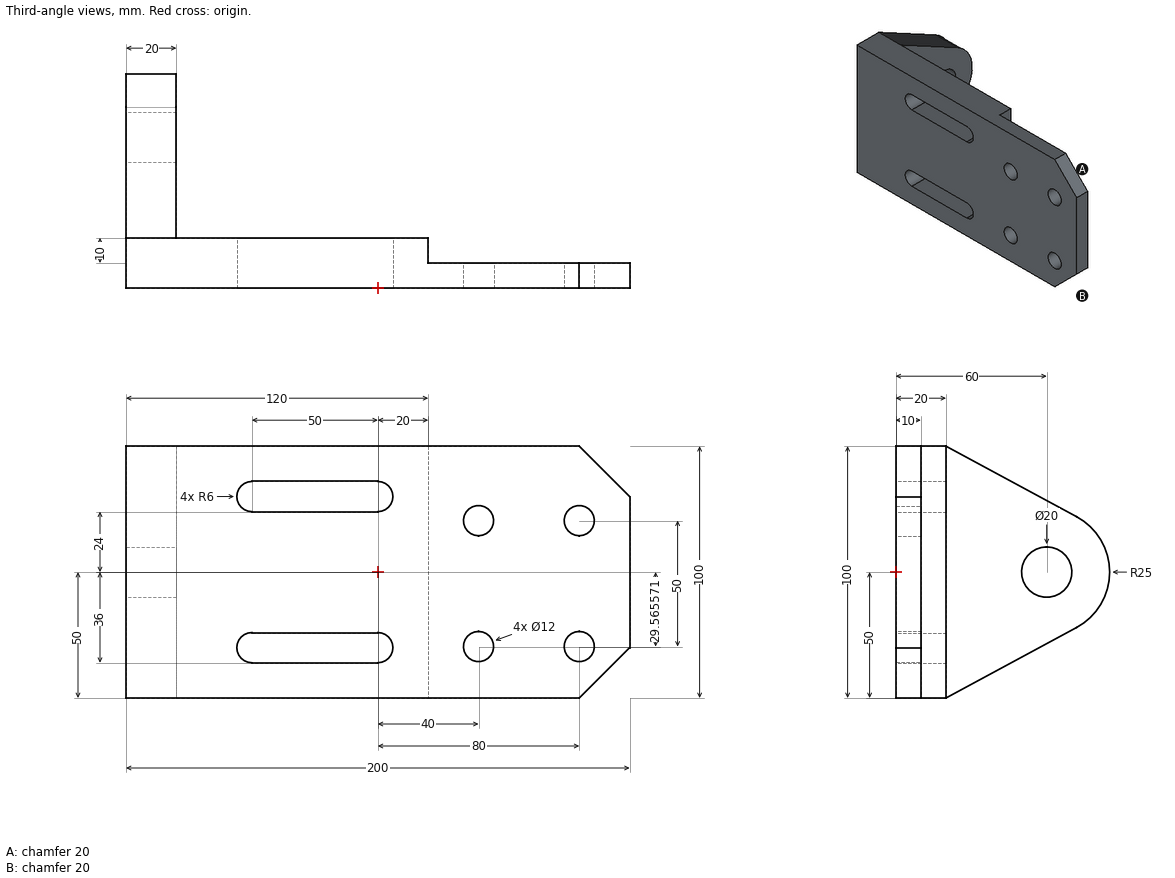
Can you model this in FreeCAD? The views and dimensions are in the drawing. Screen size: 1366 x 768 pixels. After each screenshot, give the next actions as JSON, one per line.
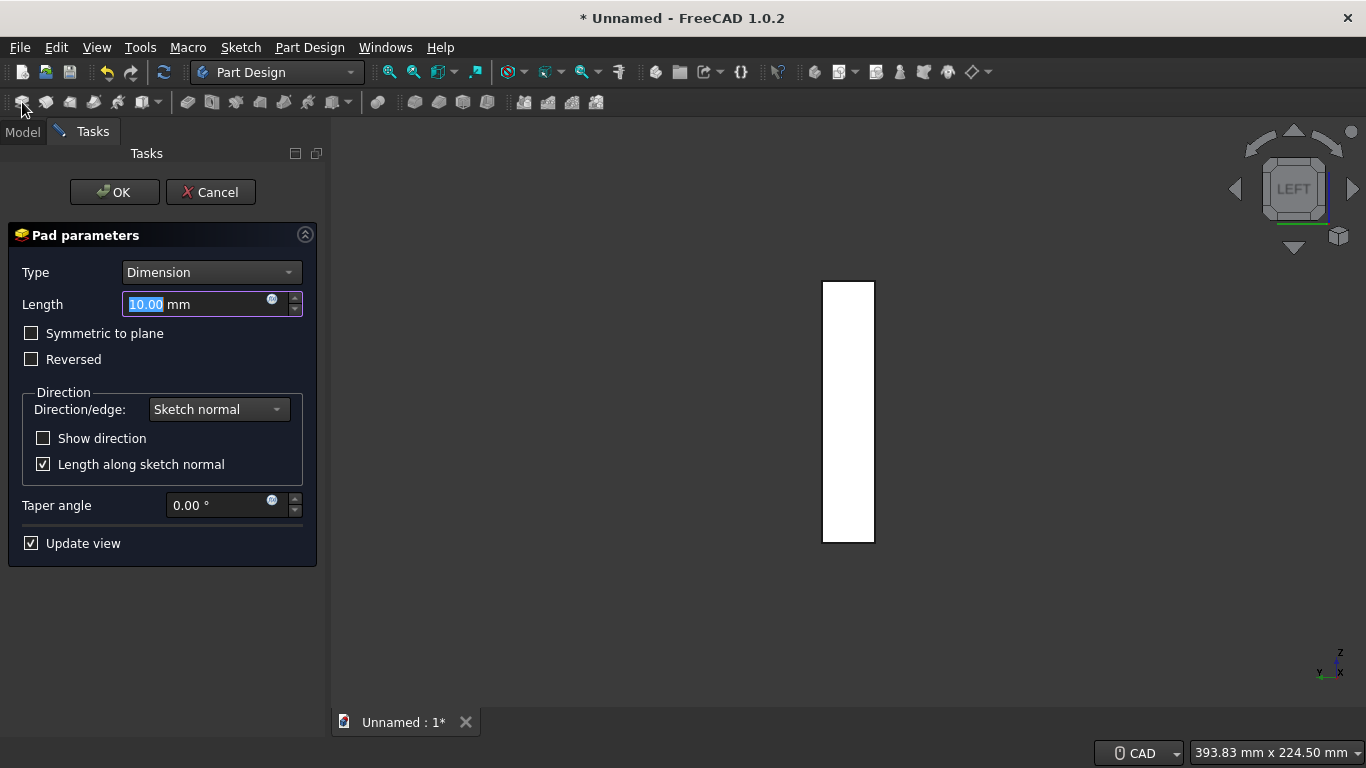
{"action": "type", "text": "20"}
{"action": "key", "text": "Tab"}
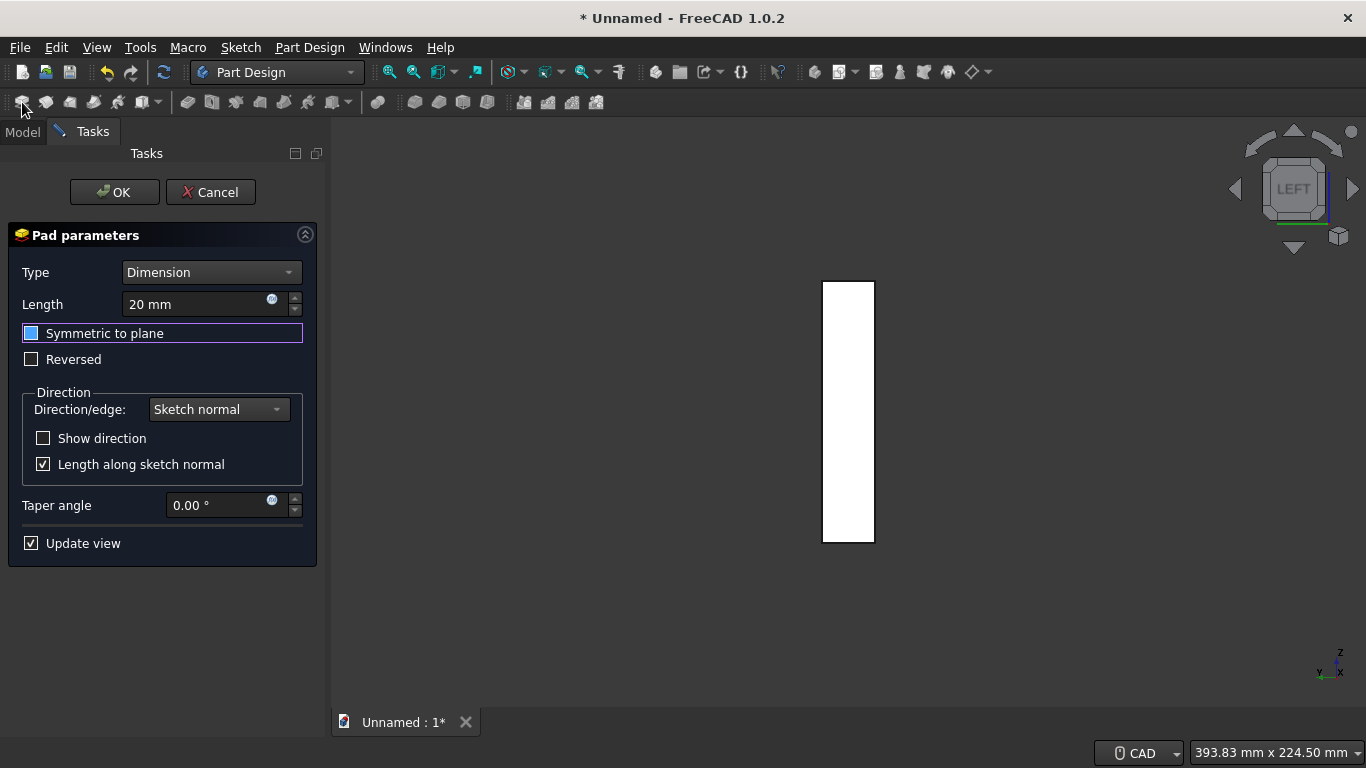
{"action": "left_click", "coordinate": [30, 359]}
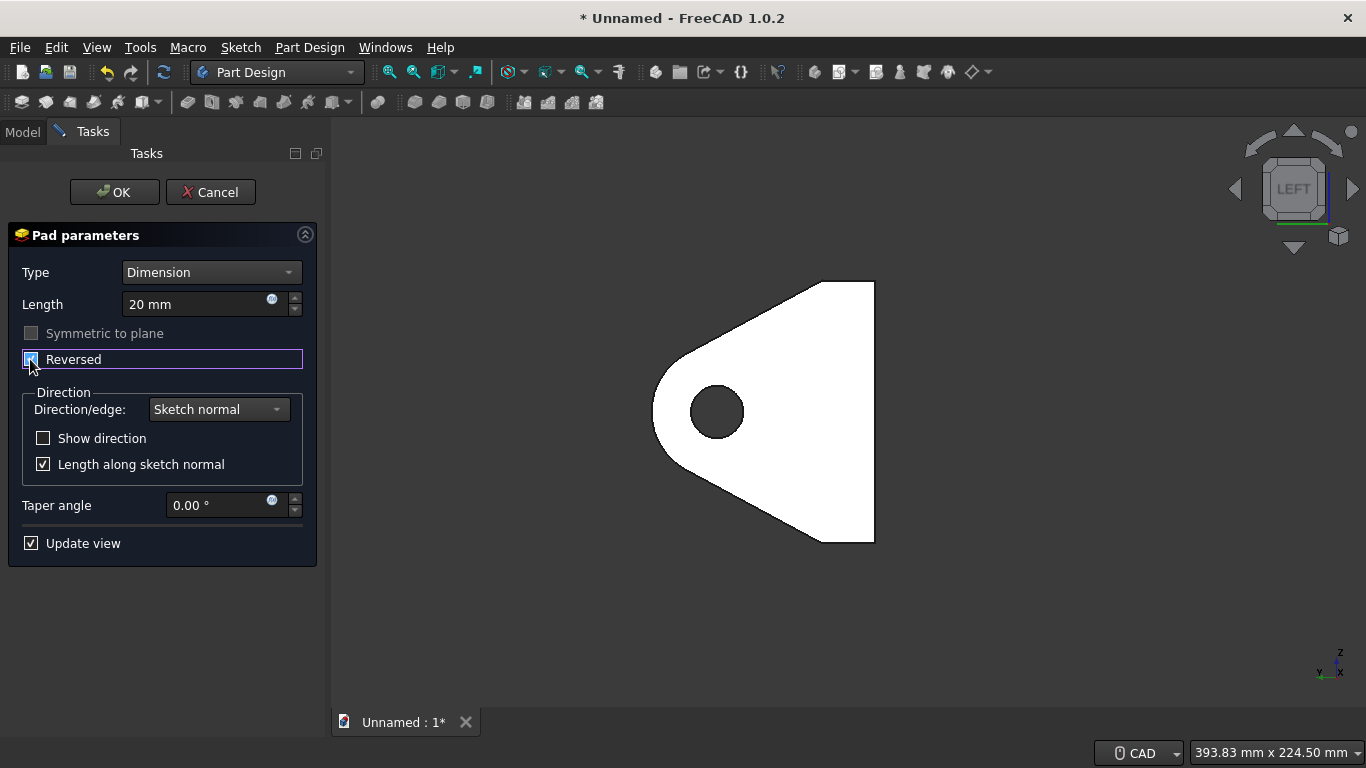
{"action": "left_click", "coordinate": [115, 192]}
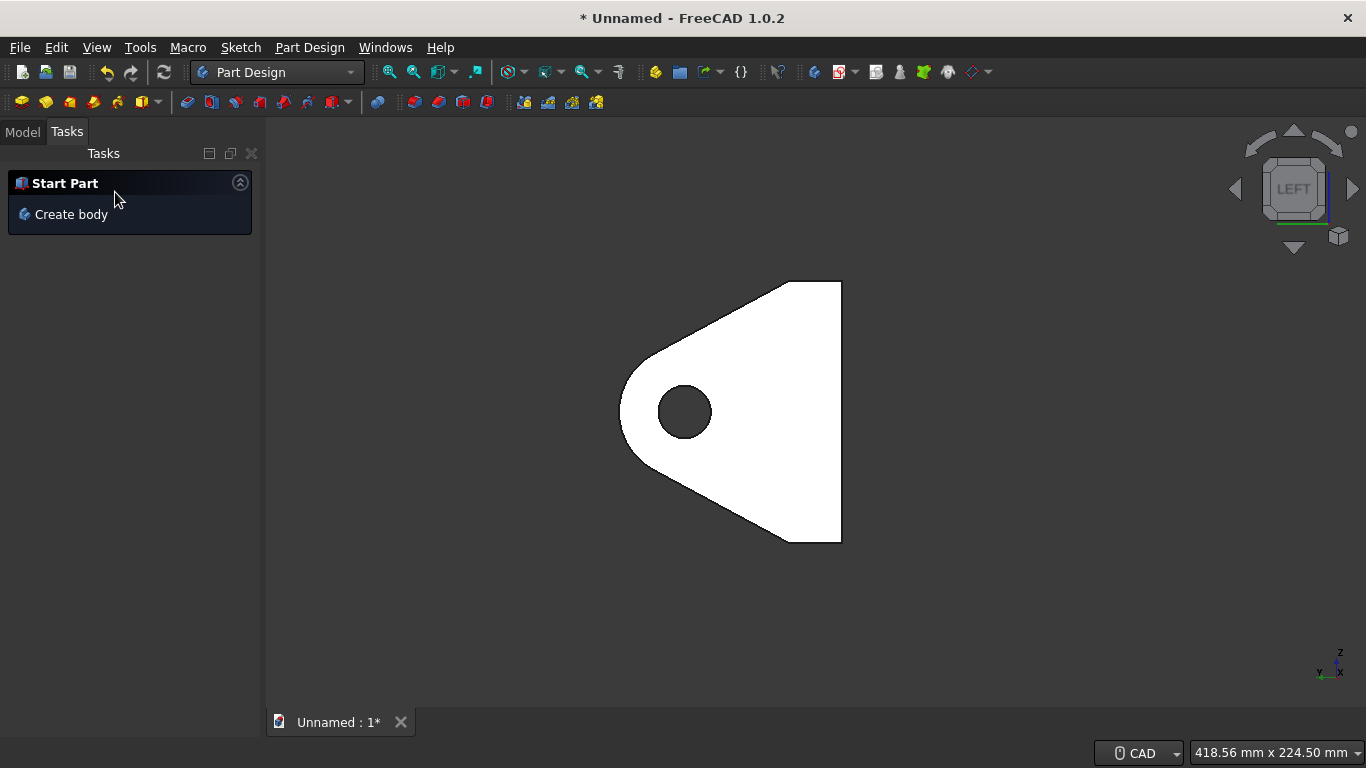
{"action": "left_click", "coordinate": [390, 72]}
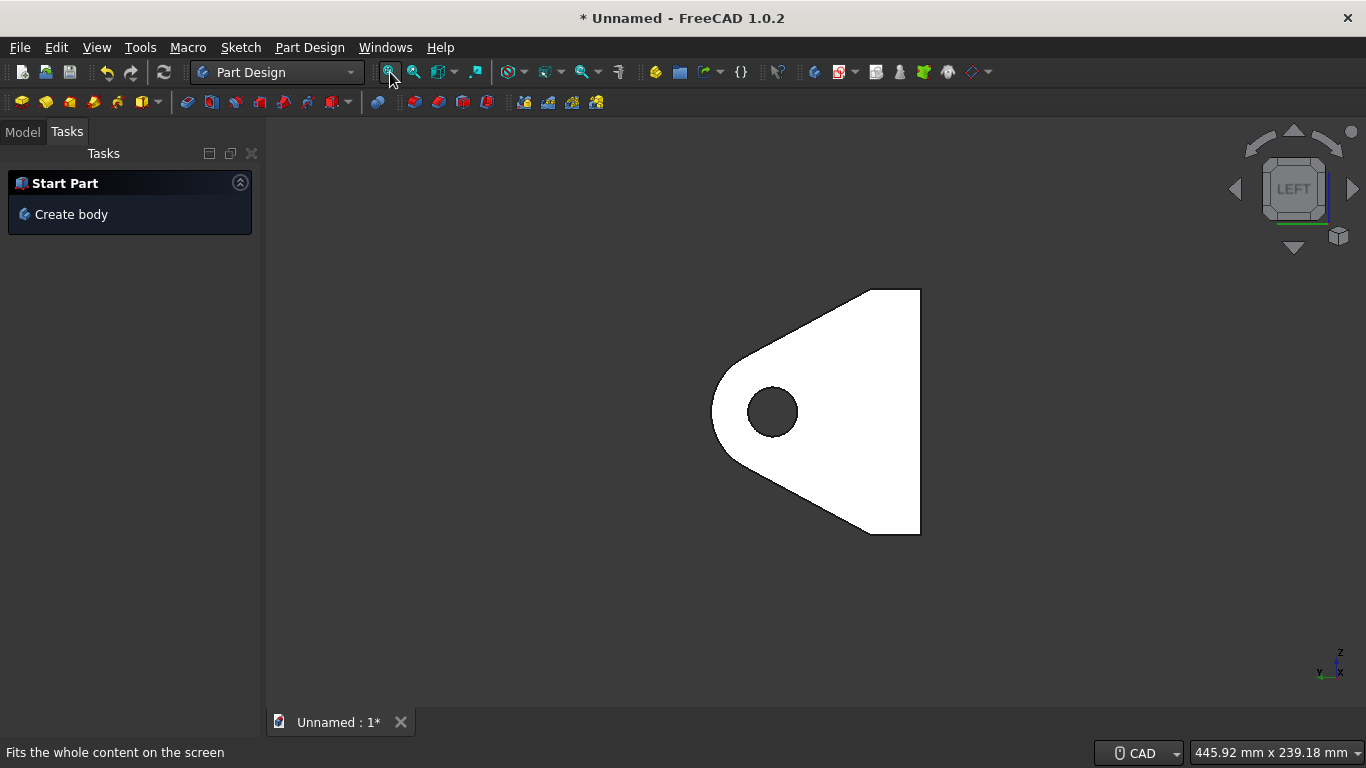
{"action": "key", "text": "4"}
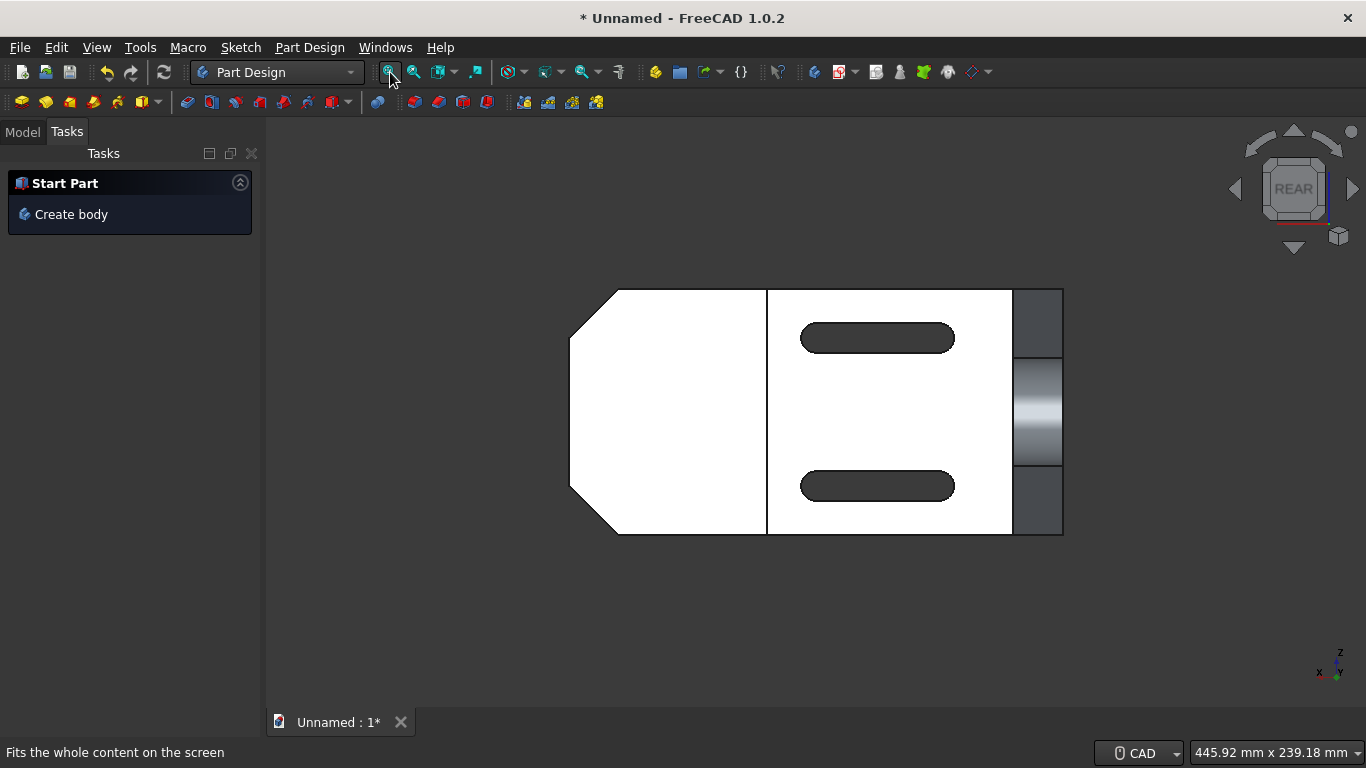
{"action": "left_click", "coordinate": [390, 72]}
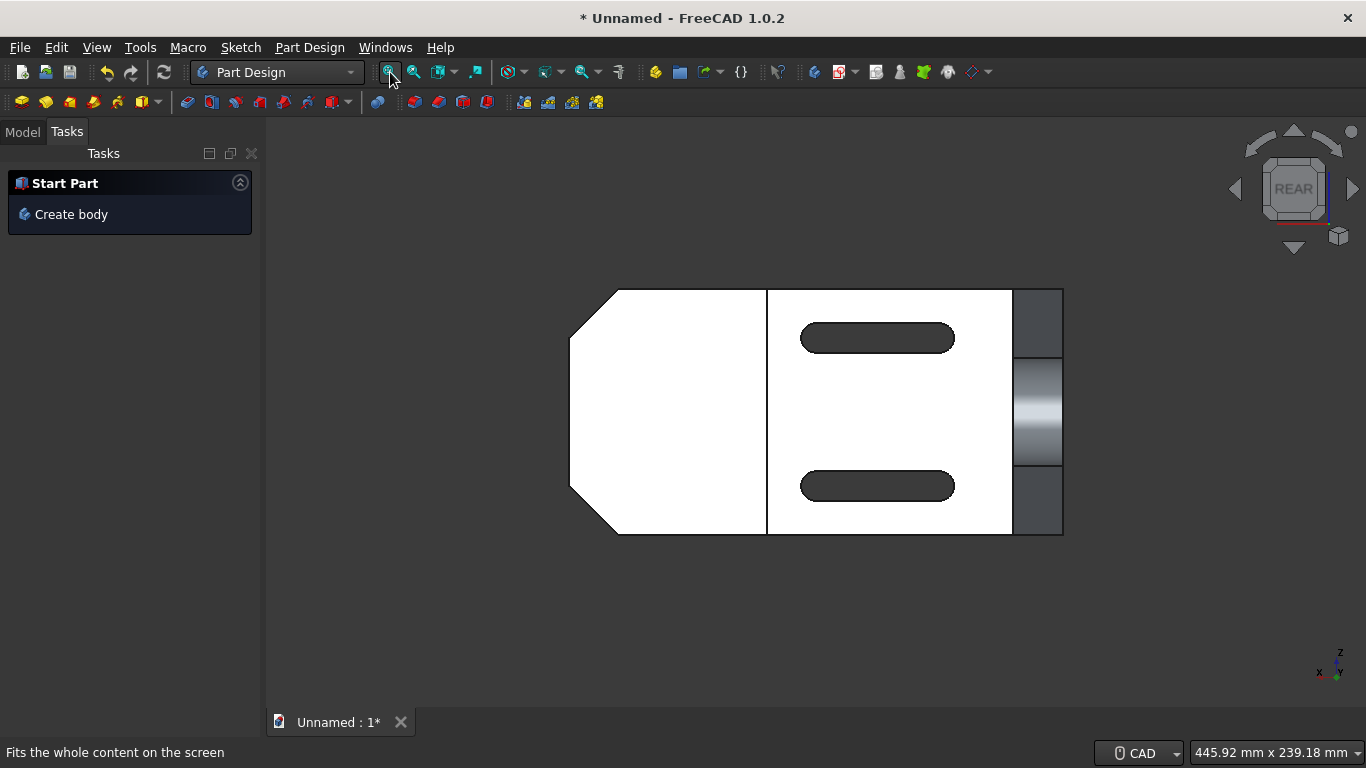
{"action": "left_click", "coordinate": [668, 411]}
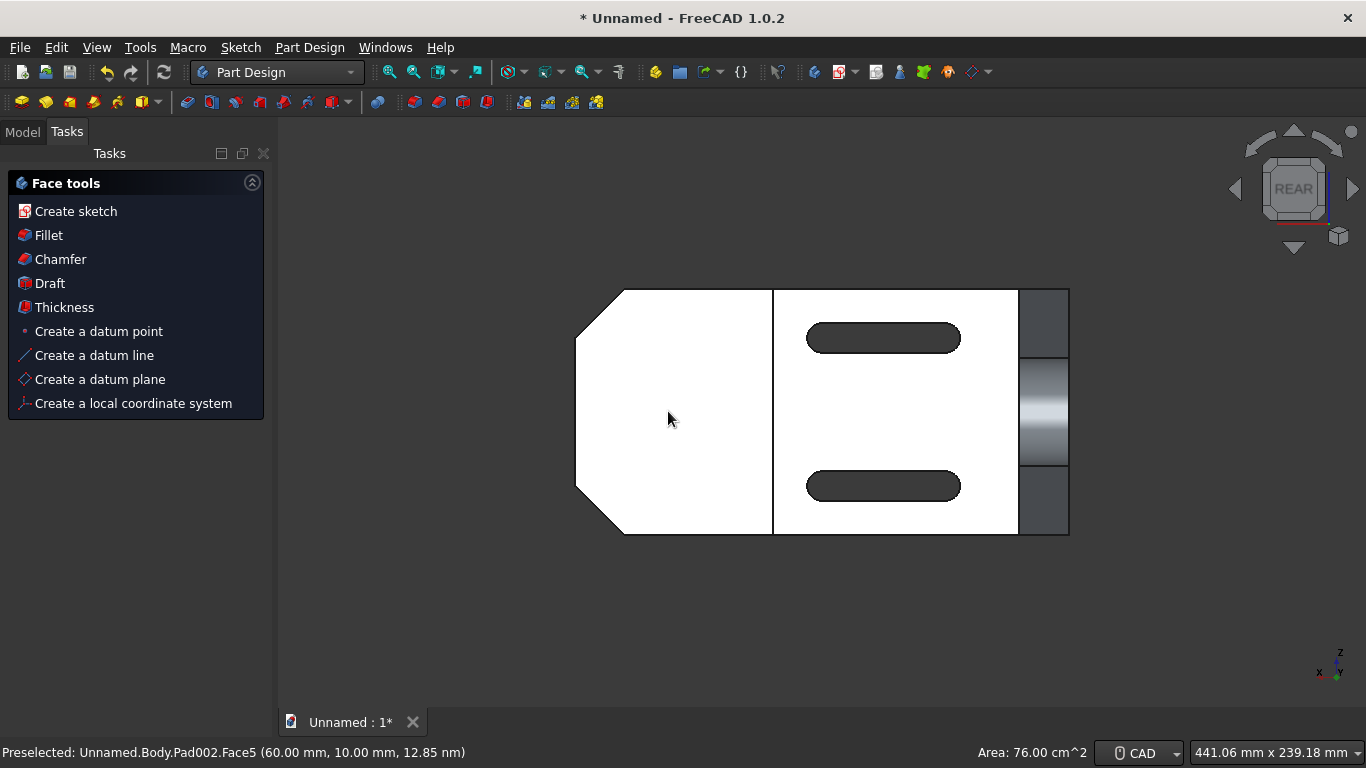
{"action": "left_click", "coordinate": [840, 72]}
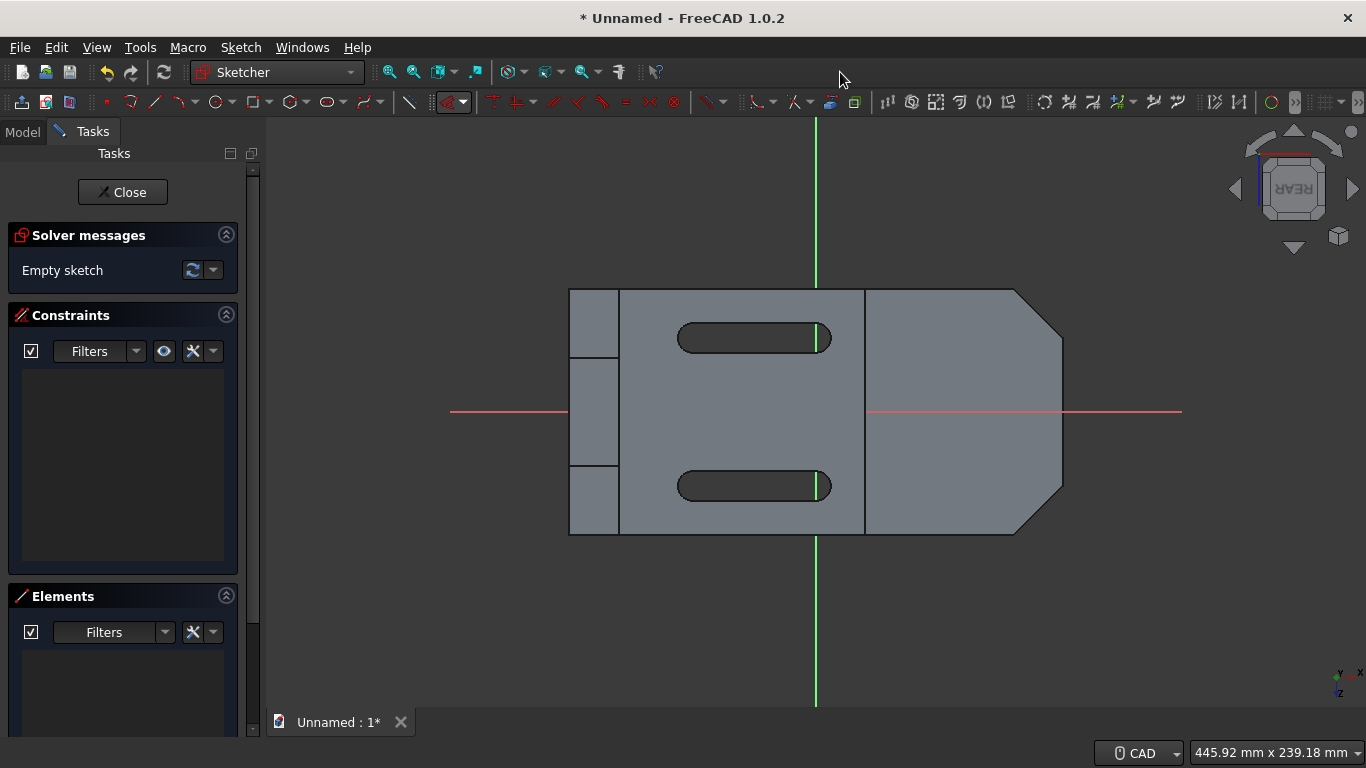
{"action": "scroll", "coordinate": [1024, 394], "scroll_direction": "up", "scroll_amount": 5}